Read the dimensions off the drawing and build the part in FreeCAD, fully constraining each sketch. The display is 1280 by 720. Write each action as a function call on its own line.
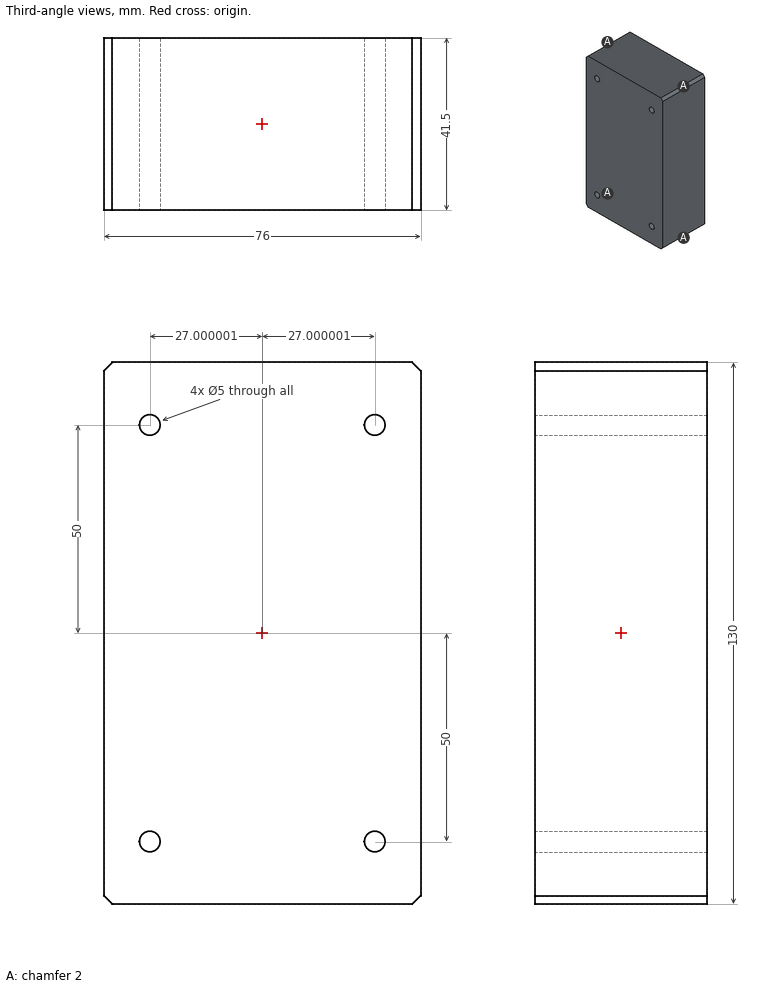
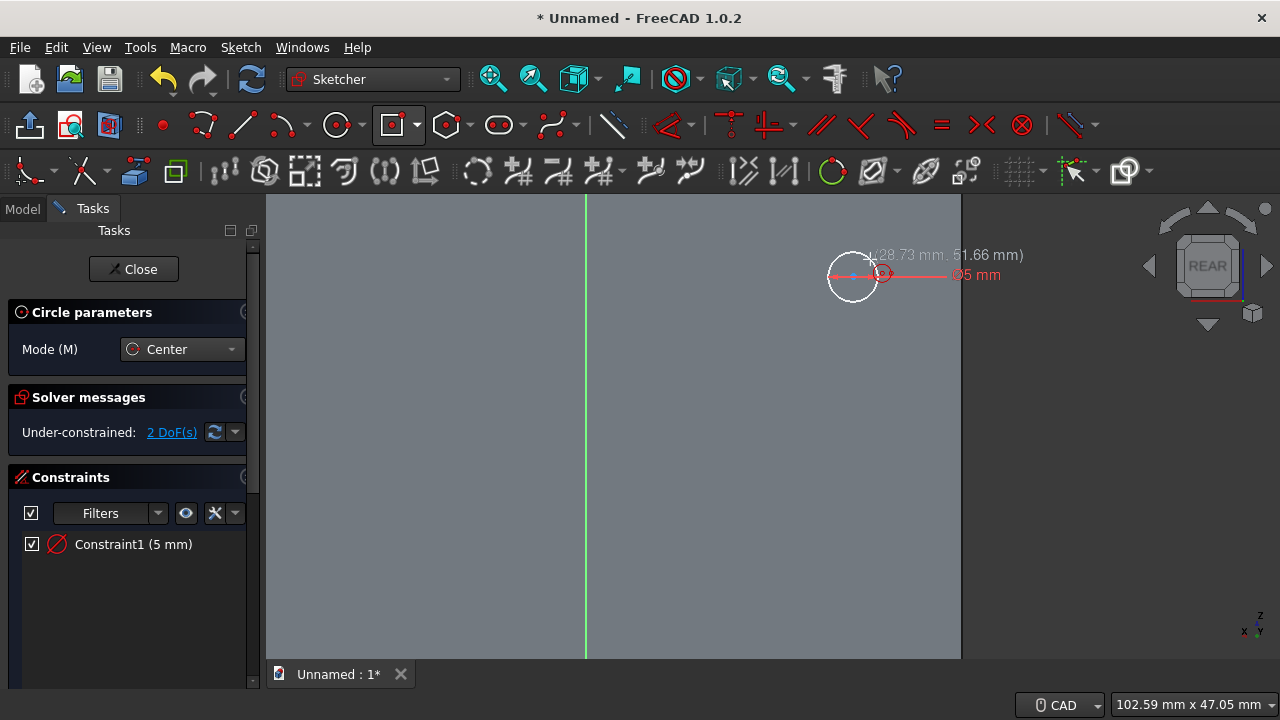
click(319, 276)
move(337, 259)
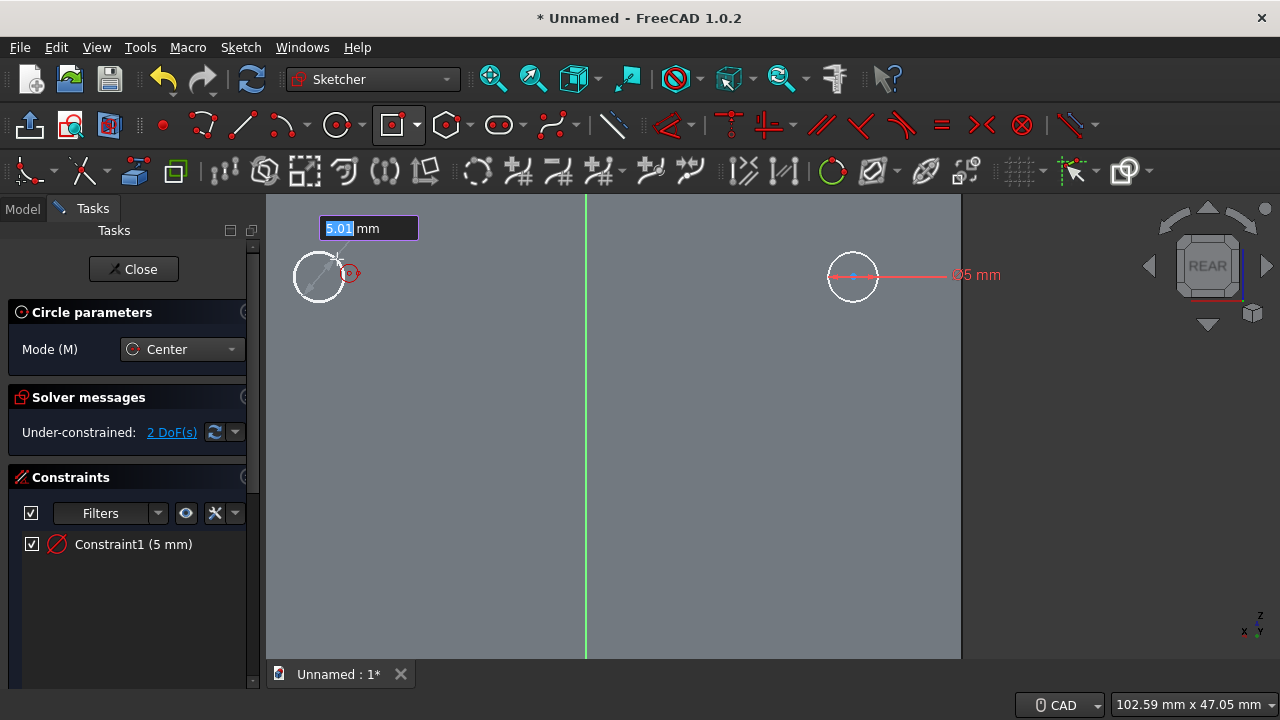
text(5)
key(Return)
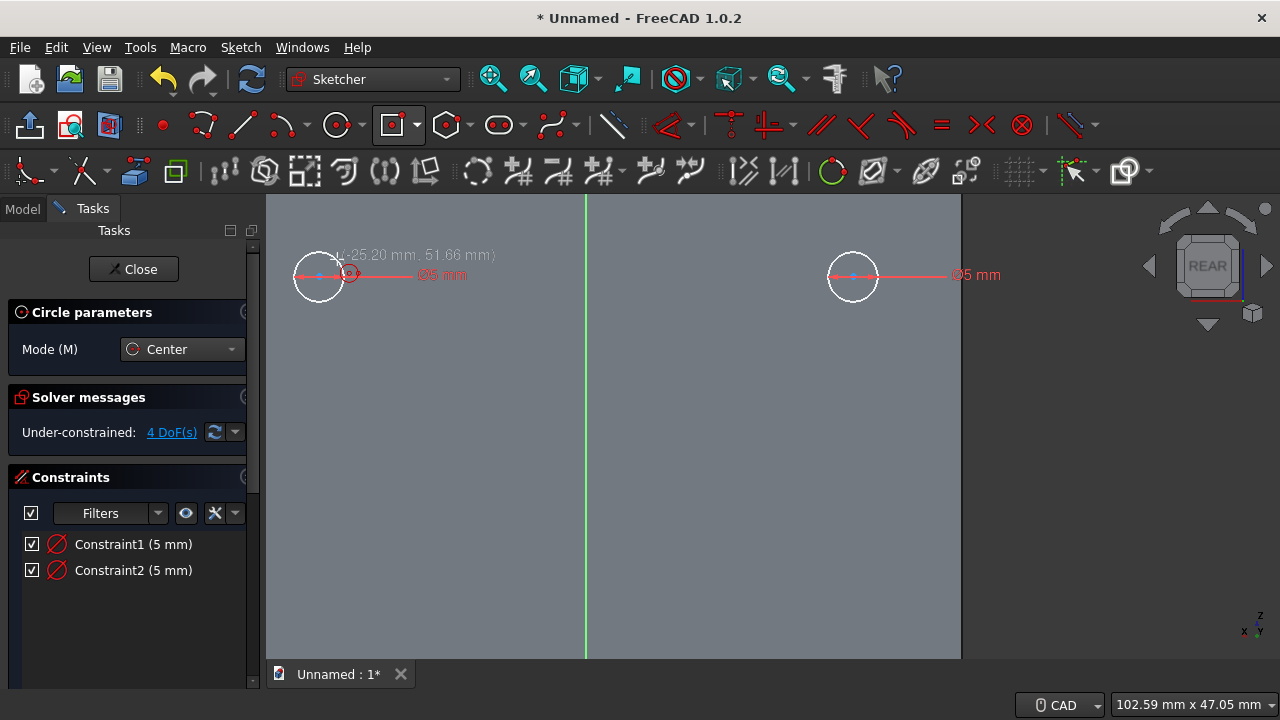
scroll(756, 278, down, 6)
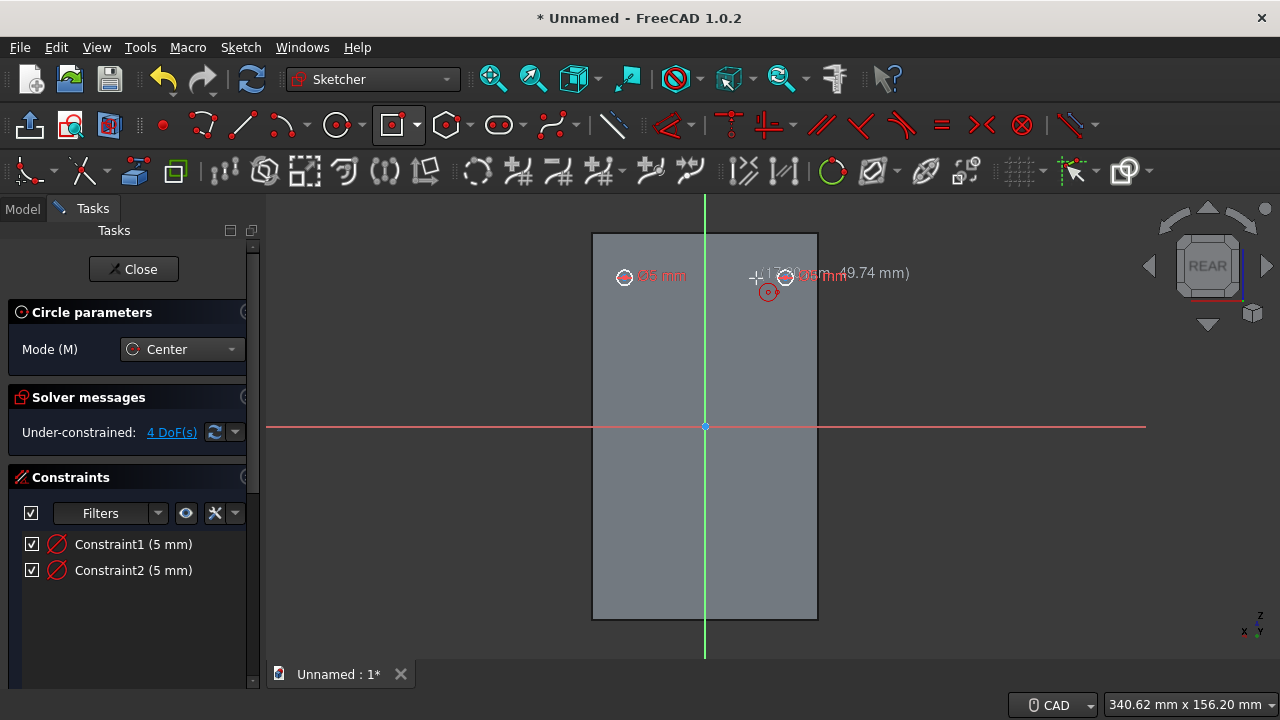
scroll(625, 575, up, 6)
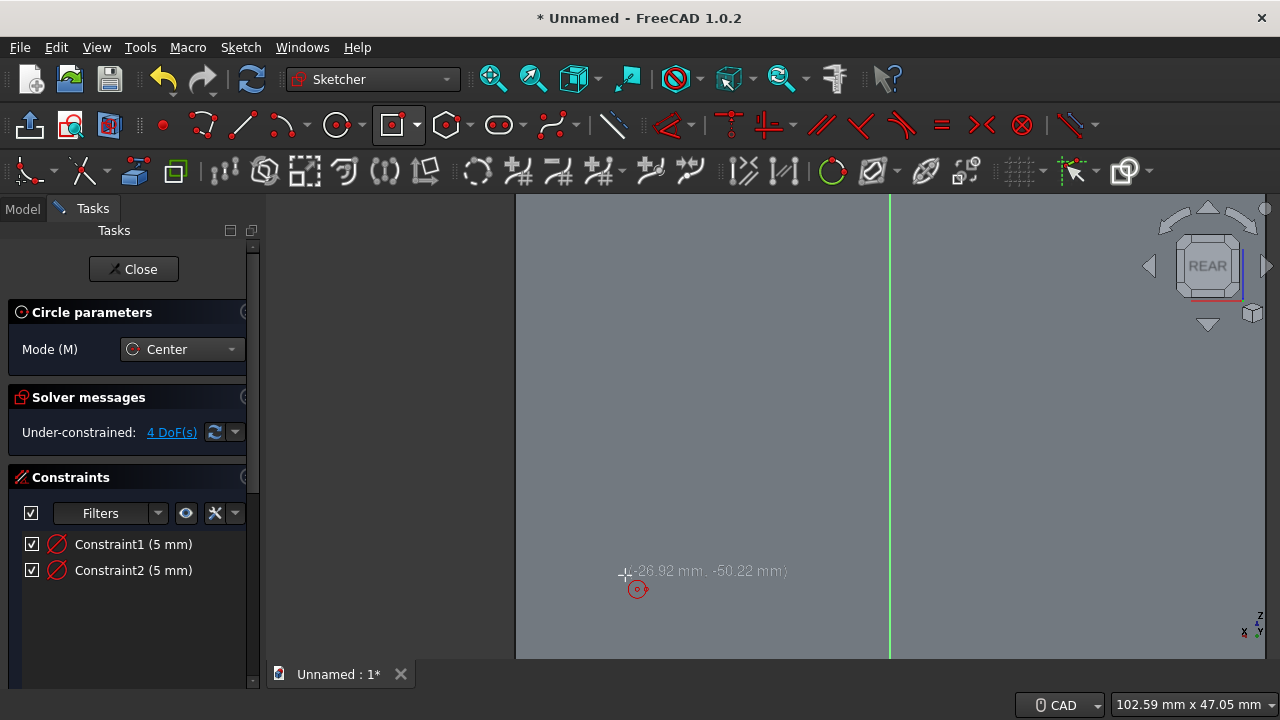
click(623, 574)
move(641, 557)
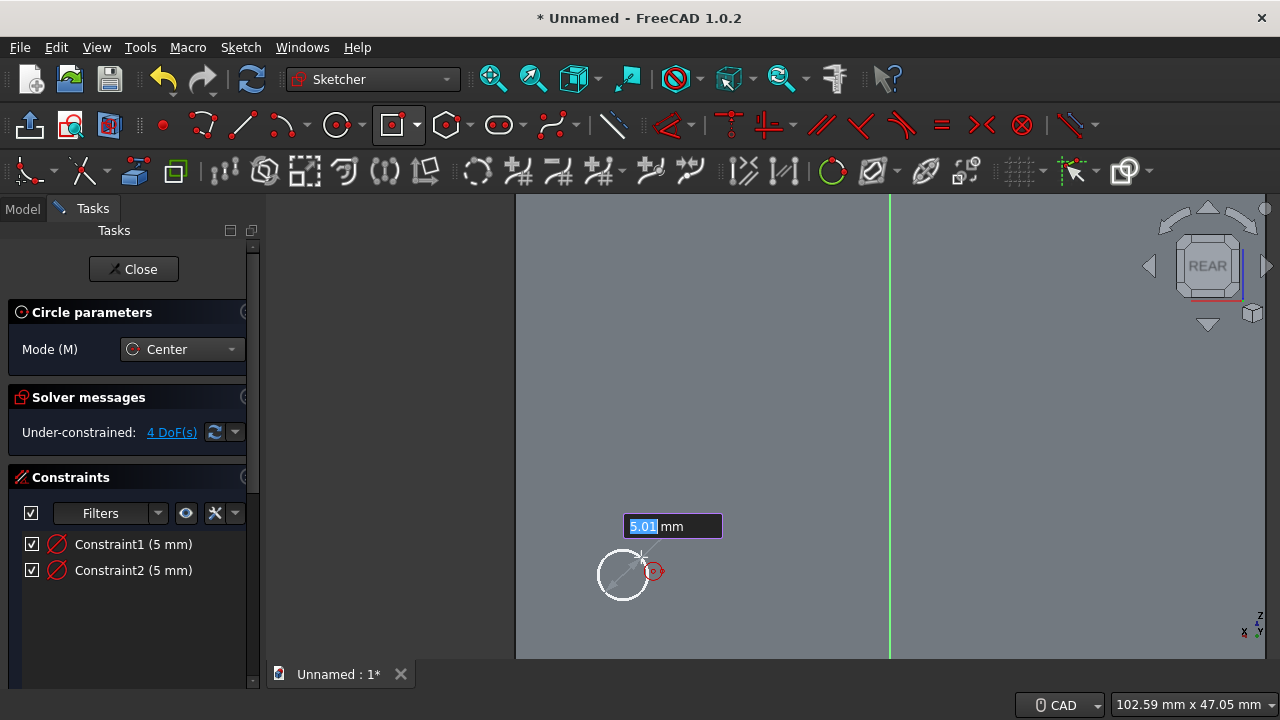
text(5)
key(Return)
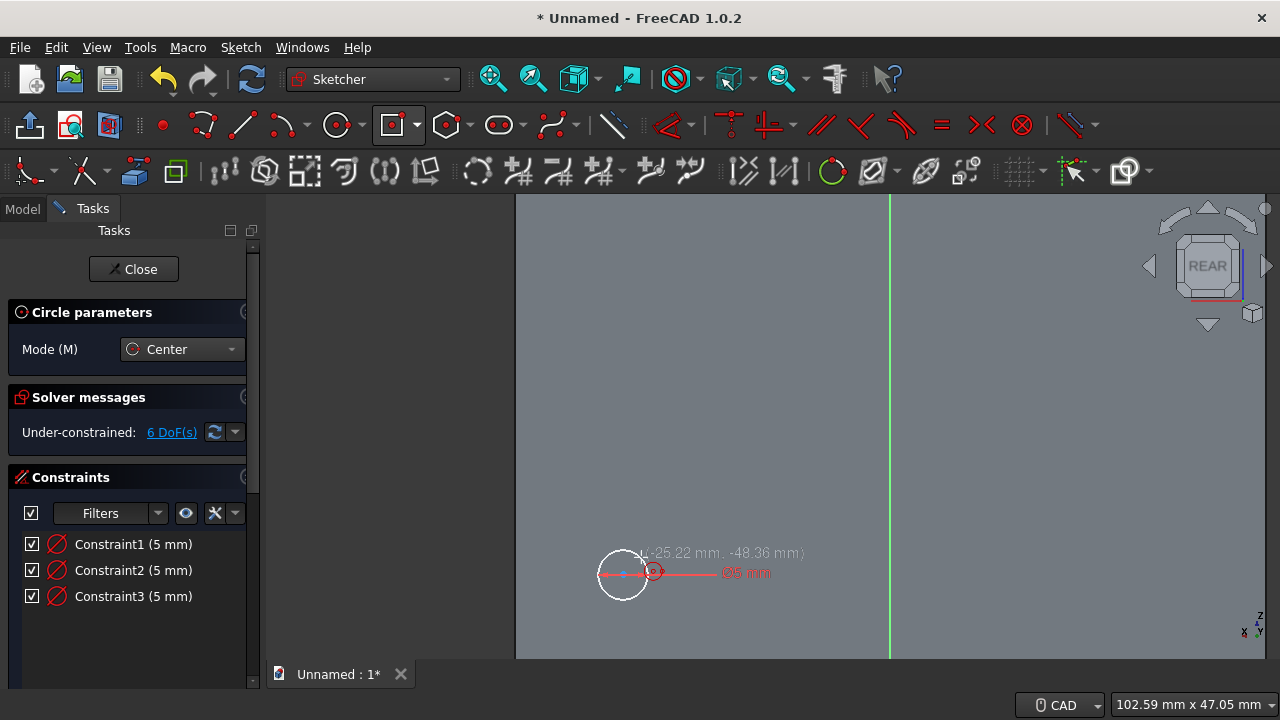
scroll(624, 576, down, 6)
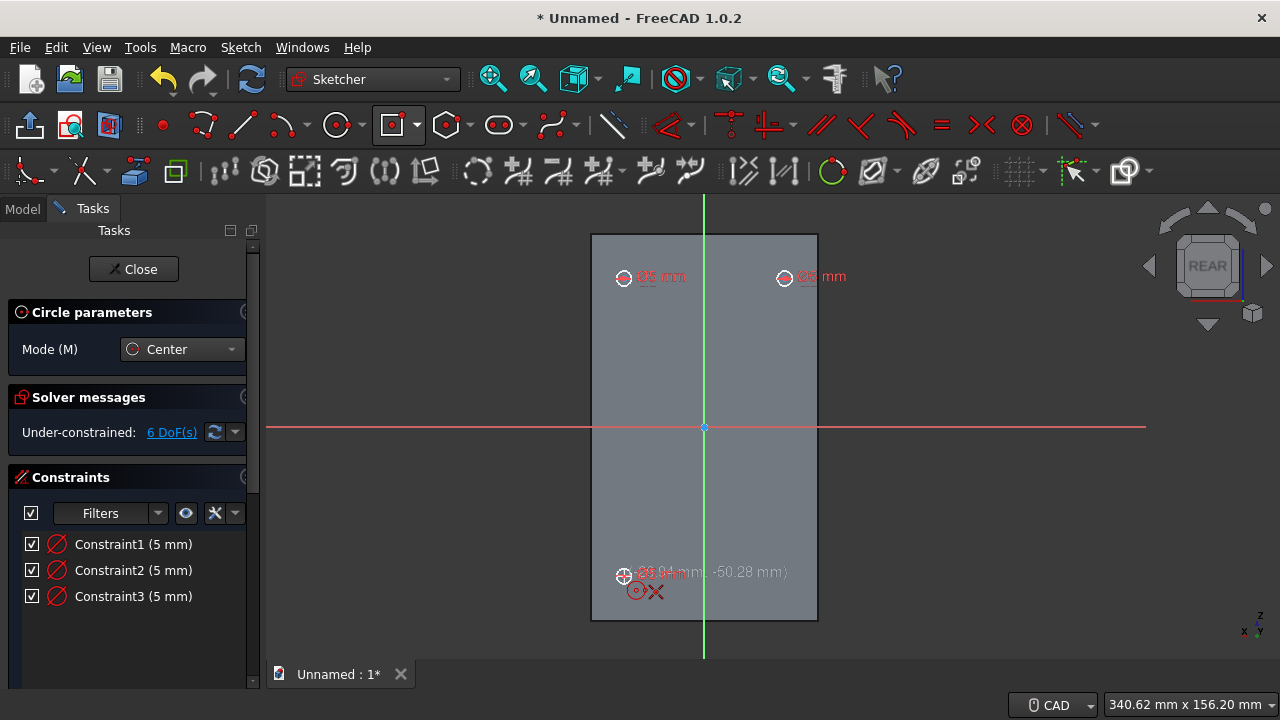
scroll(785, 576, up, 6)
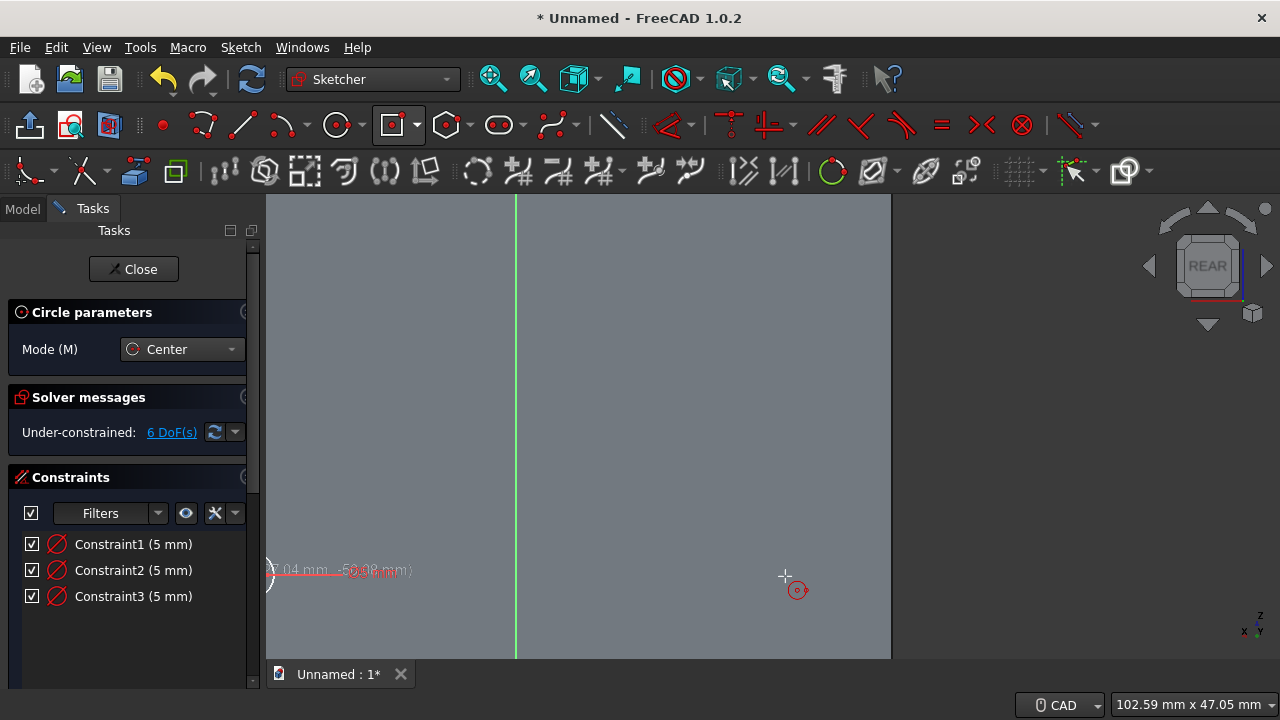
click(783, 574)
move(801, 557)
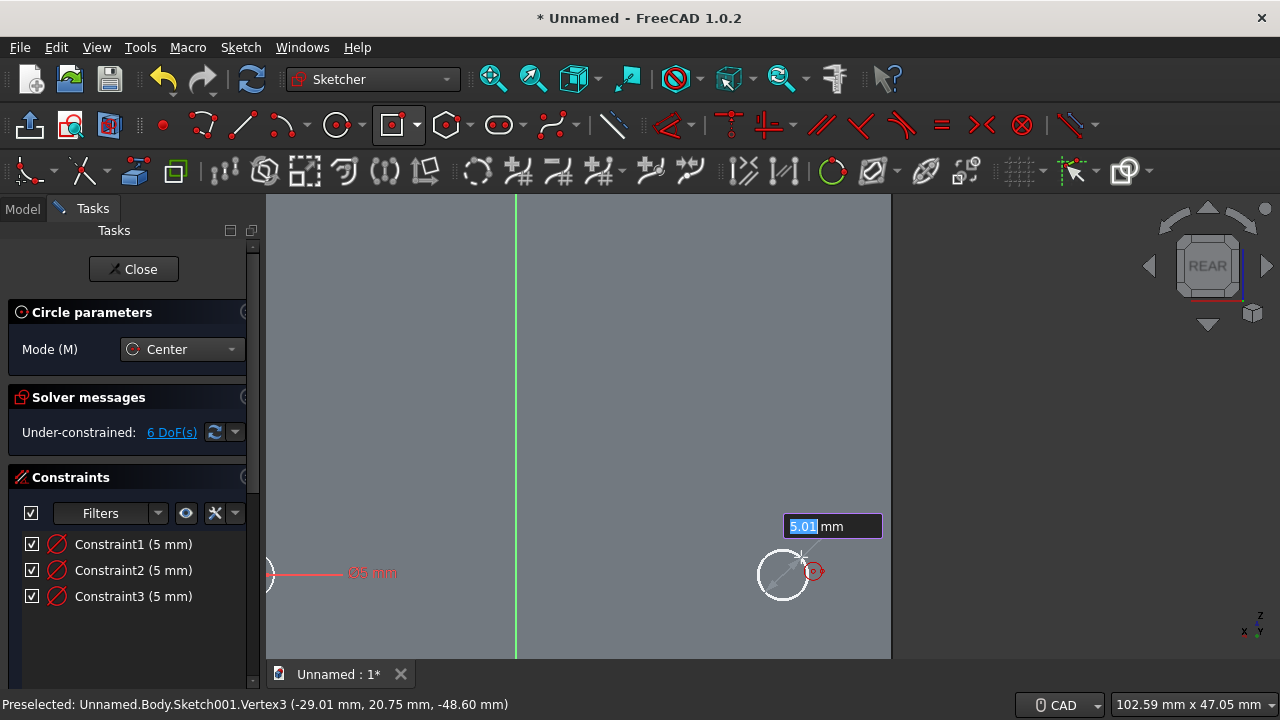
text(5)
key(Return)
key(Escape)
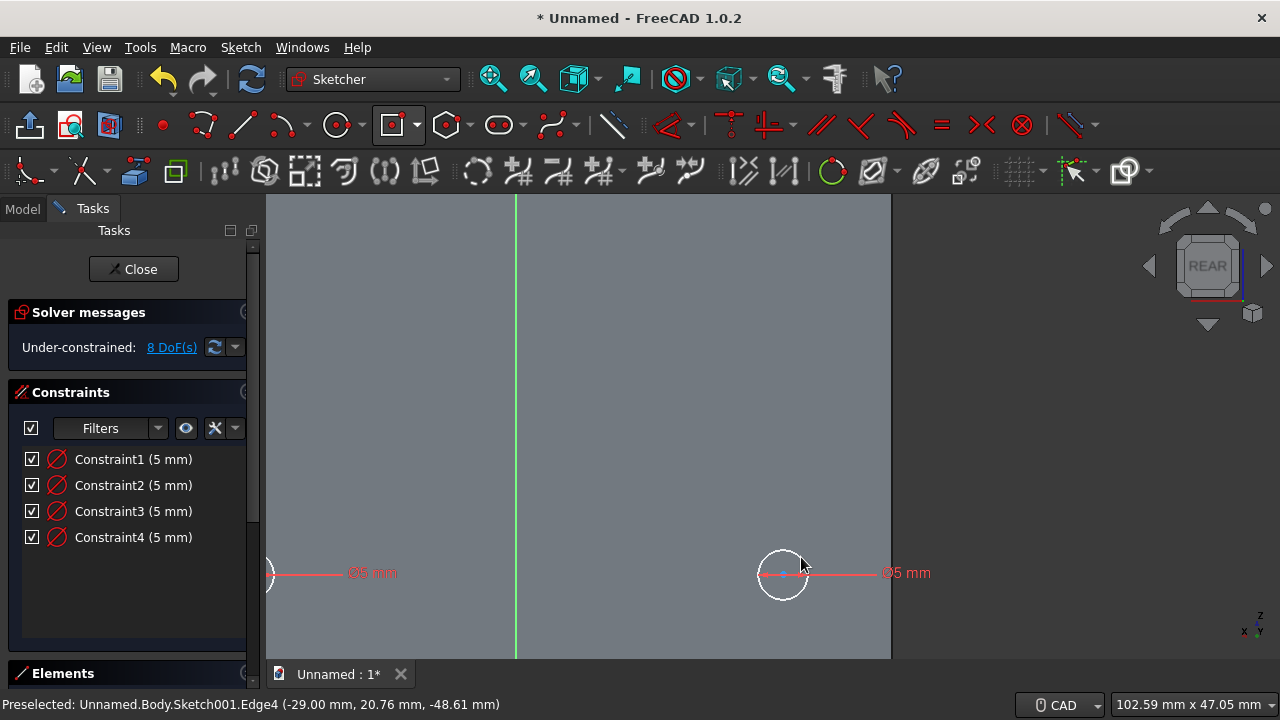
scroll(786, 576, down, 6)